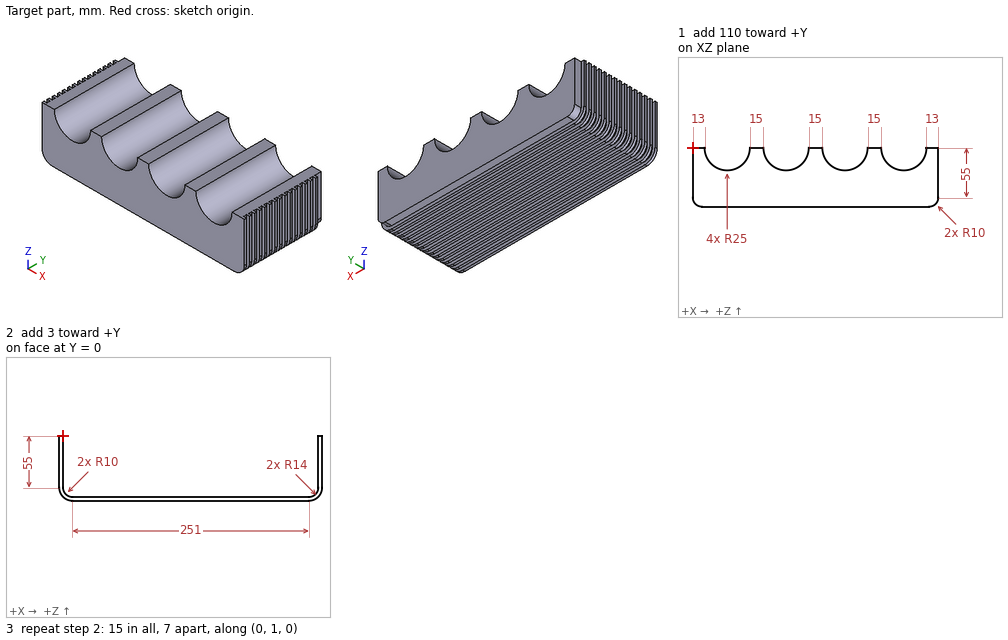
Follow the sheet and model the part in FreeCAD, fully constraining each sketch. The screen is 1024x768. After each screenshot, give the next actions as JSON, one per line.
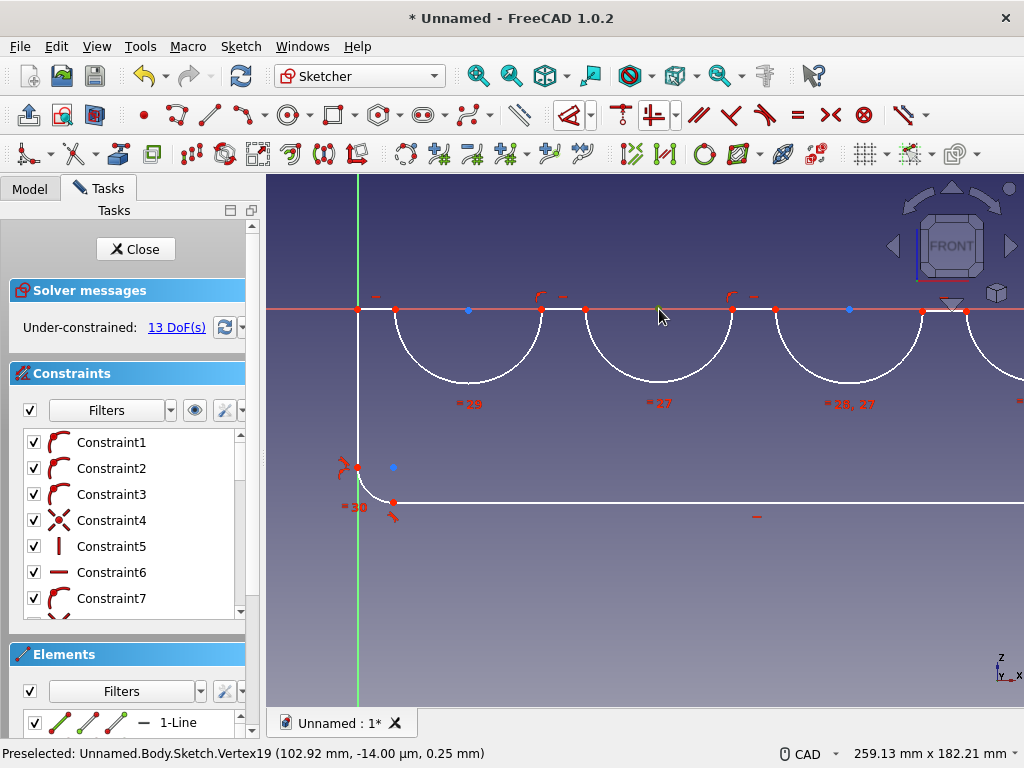
{"action": "left_click", "coordinate": [455, 309]}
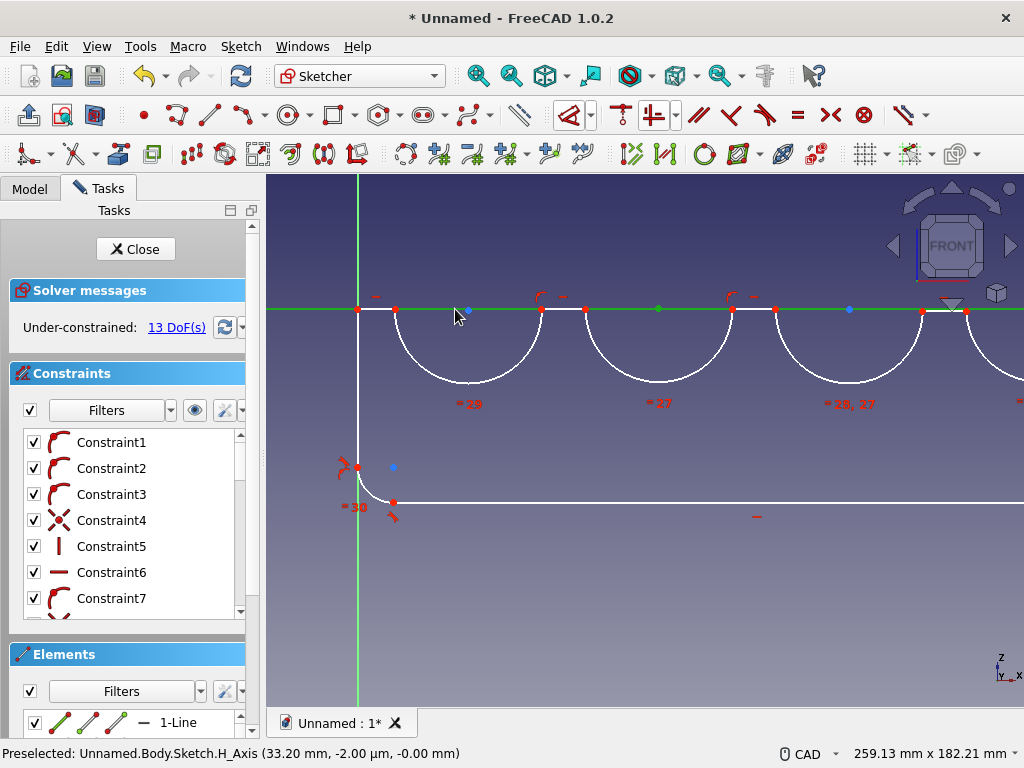
{"action": "left_click", "coordinate": [621, 116]}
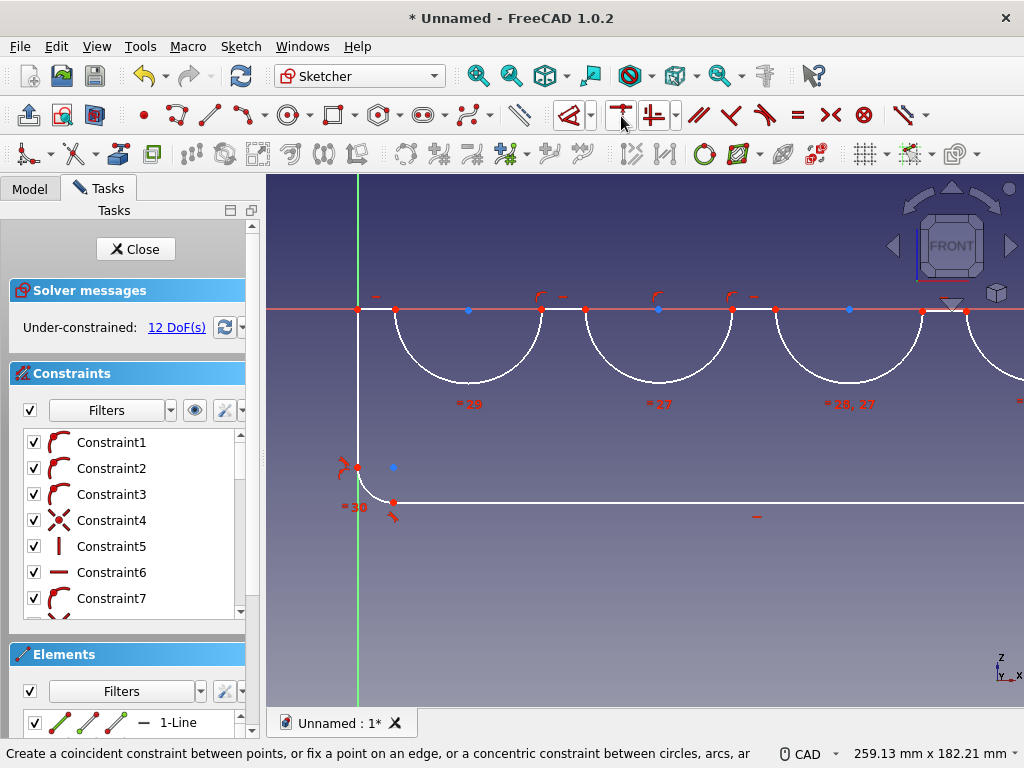
{"action": "left_click", "coordinate": [849, 310]}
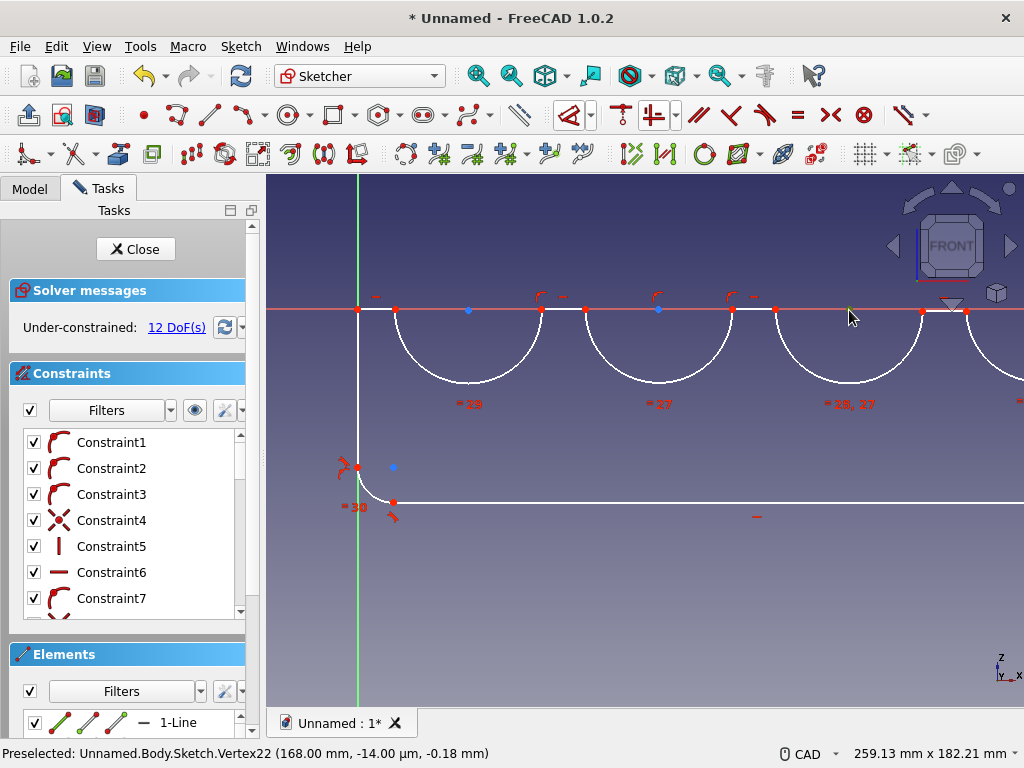
{"action": "left_click", "coordinate": [455, 309]}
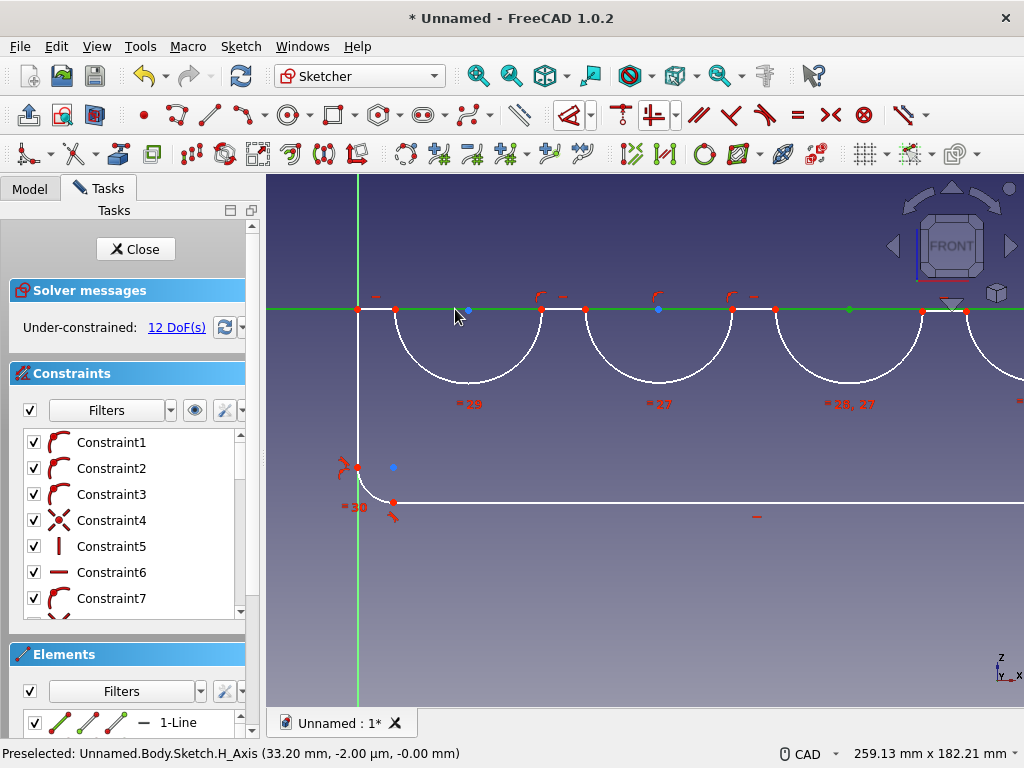
{"action": "left_click", "coordinate": [621, 116]}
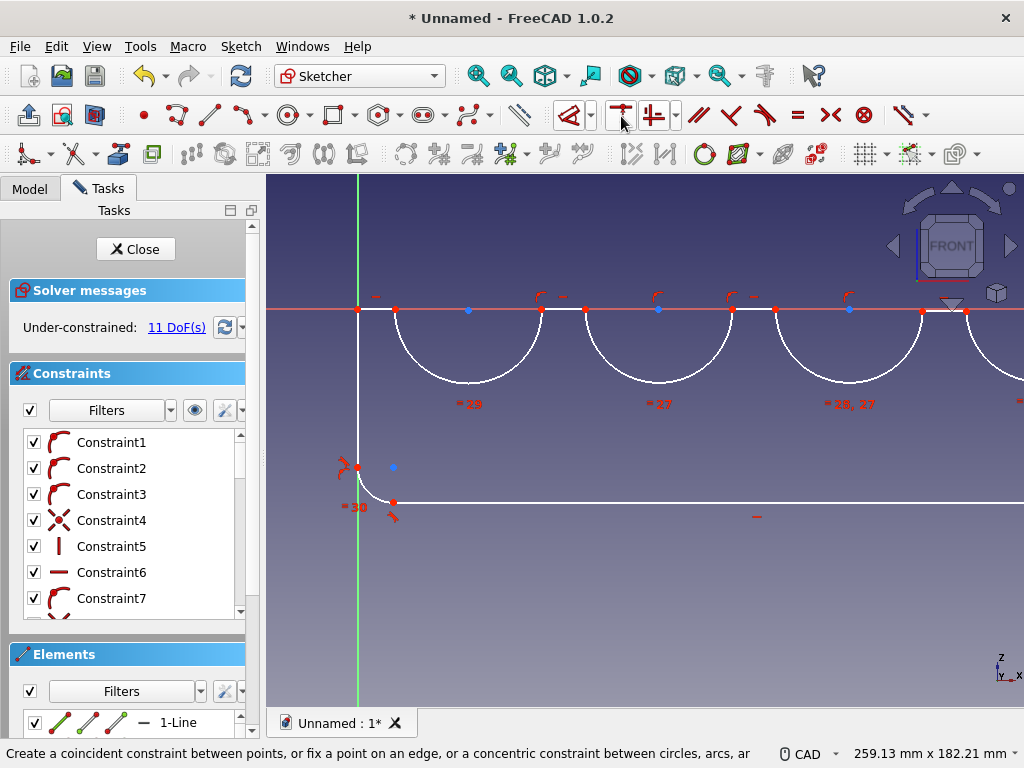
{"action": "scroll", "coordinate": [360, 484], "scroll_direction": "down", "scroll_amount": 3}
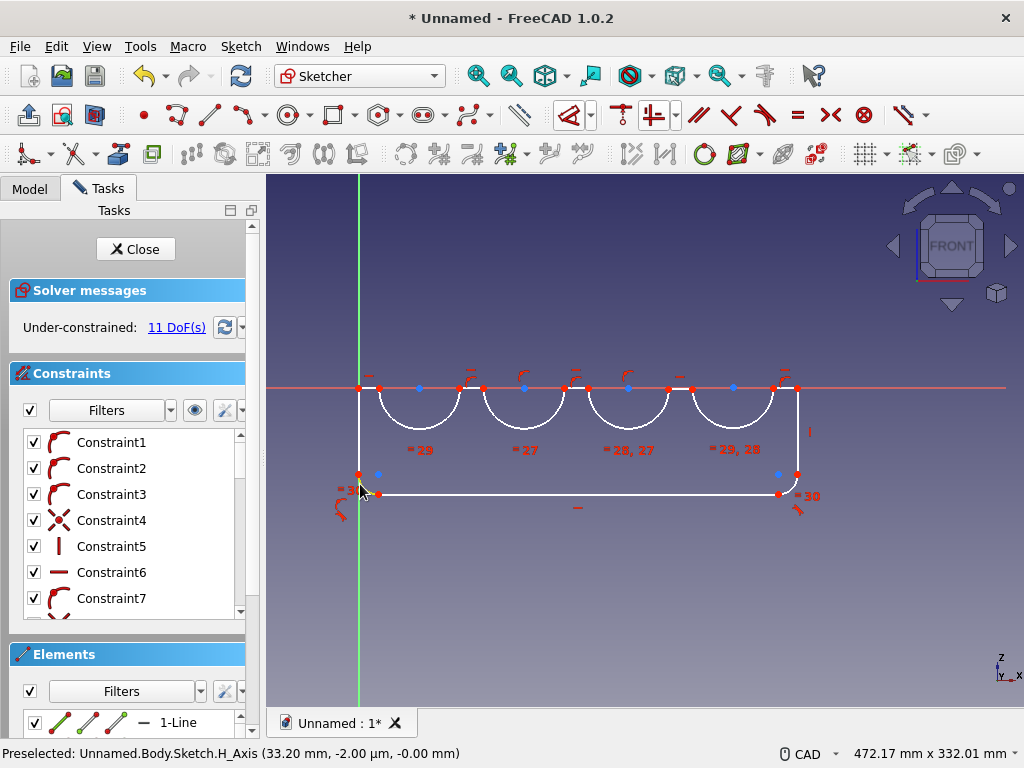
{"action": "left_click", "coordinate": [733, 388]}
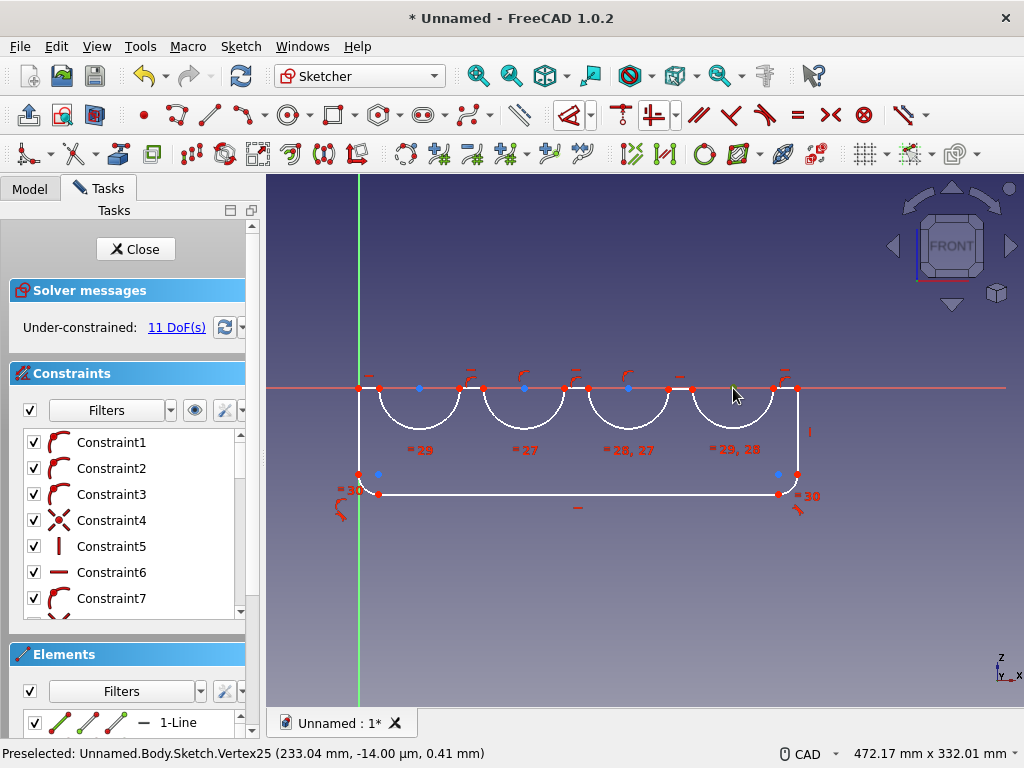
{"action": "left_click", "coordinate": [738, 388]}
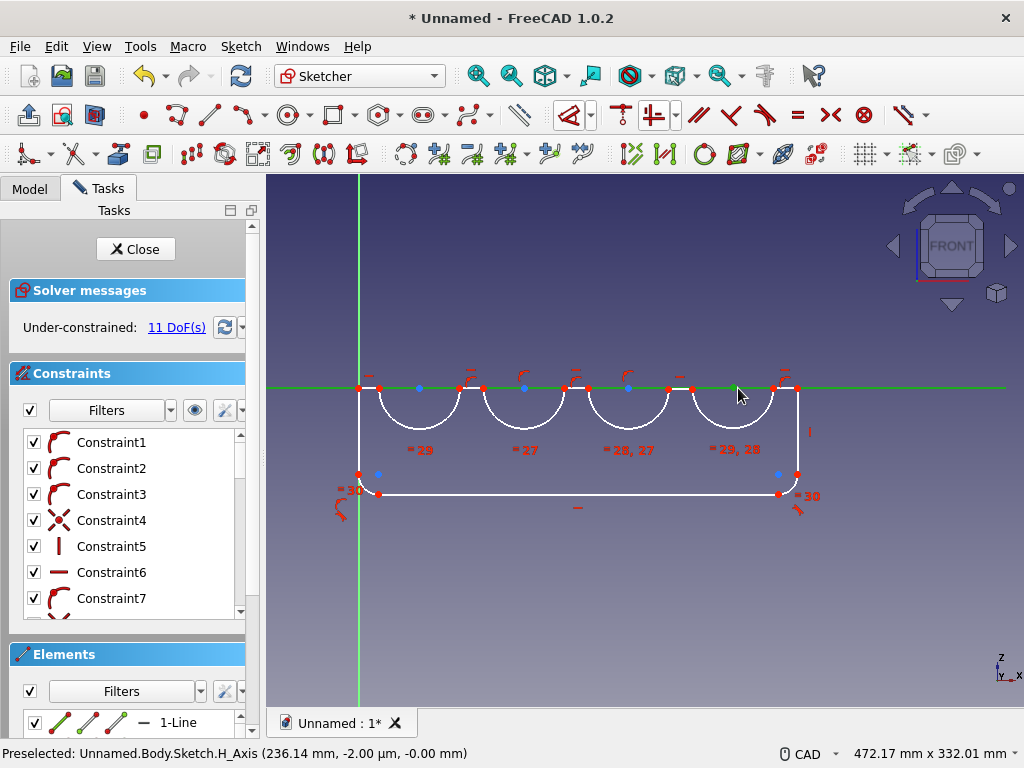
{"action": "left_click", "coordinate": [621, 116]}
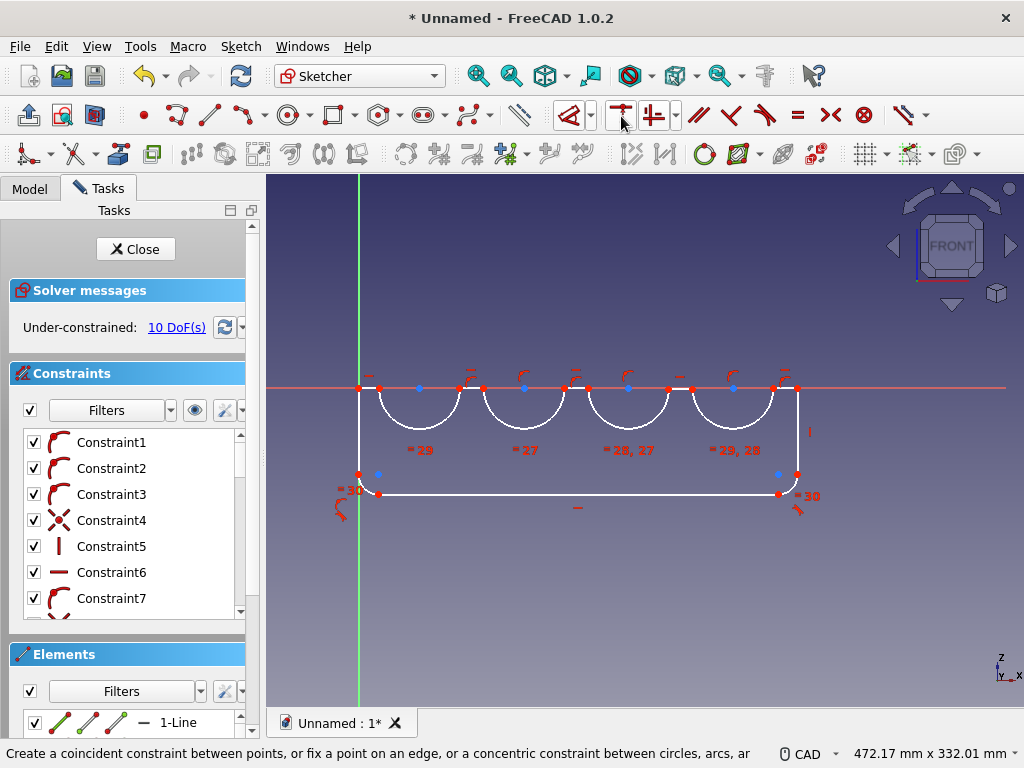
{"action": "left_click", "coordinate": [420, 389]}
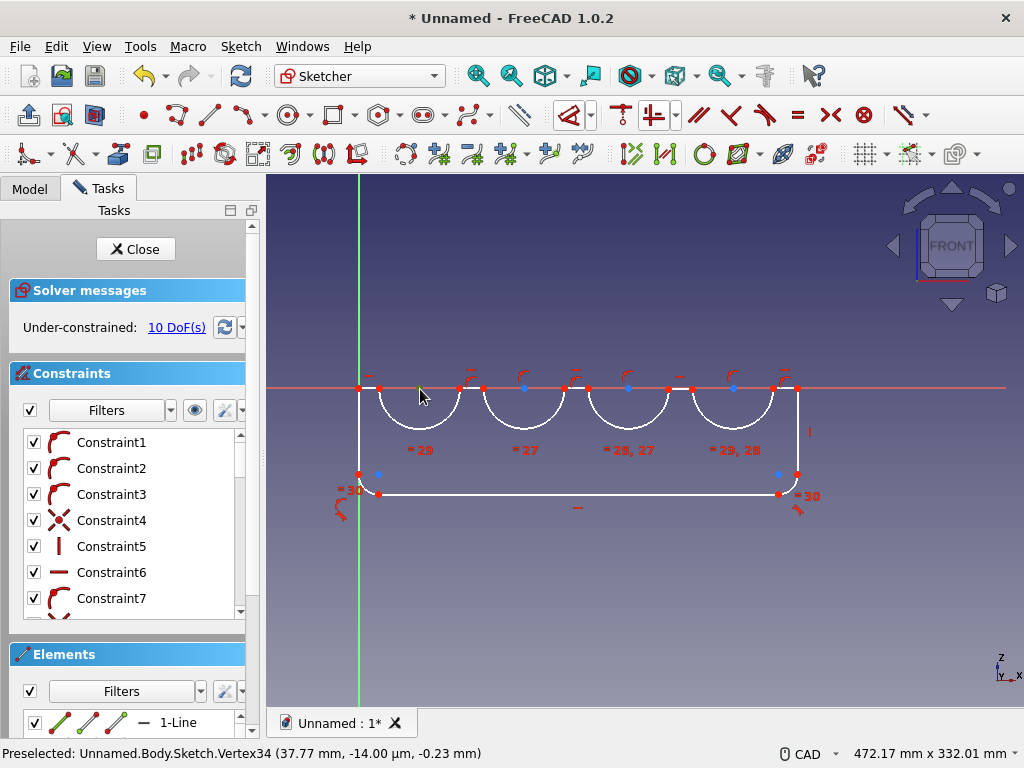
{"action": "left_click", "coordinate": [738, 388]}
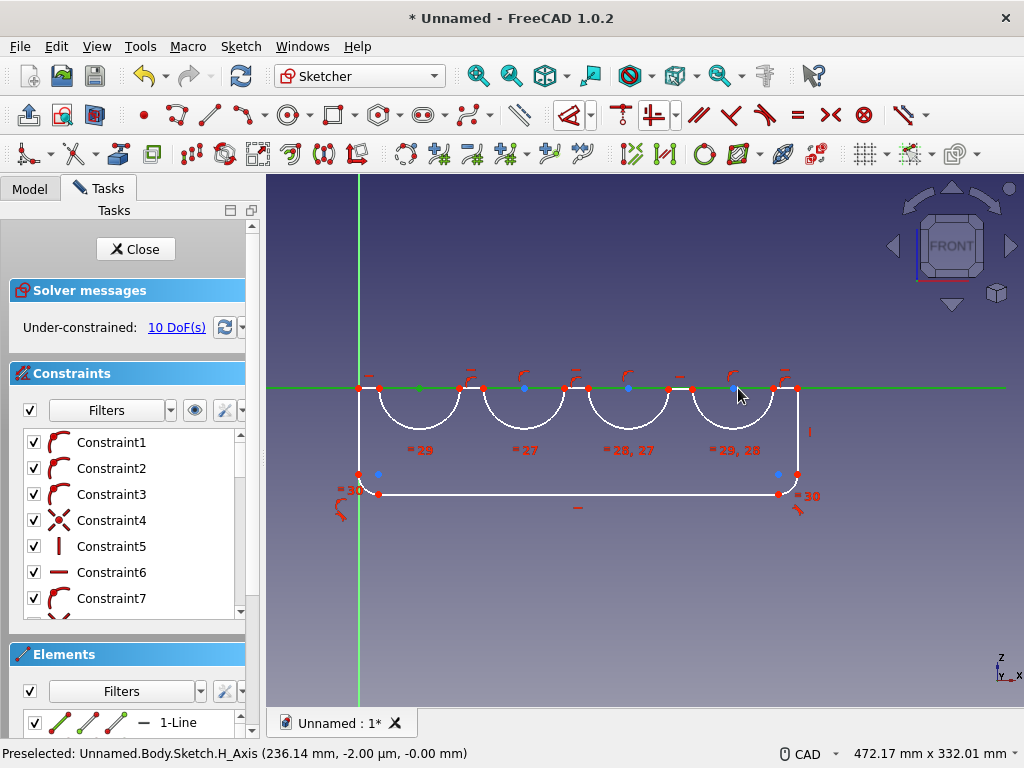
{"action": "left_click", "coordinate": [621, 116]}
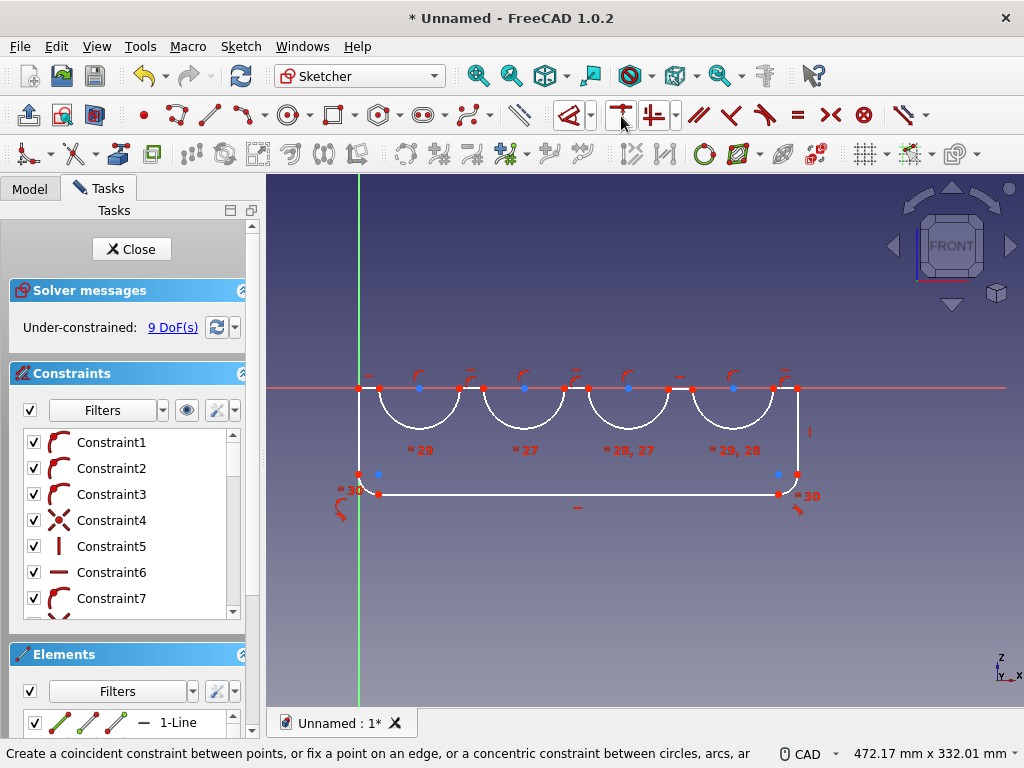
{"action": "left_click", "coordinate": [500, 421]}